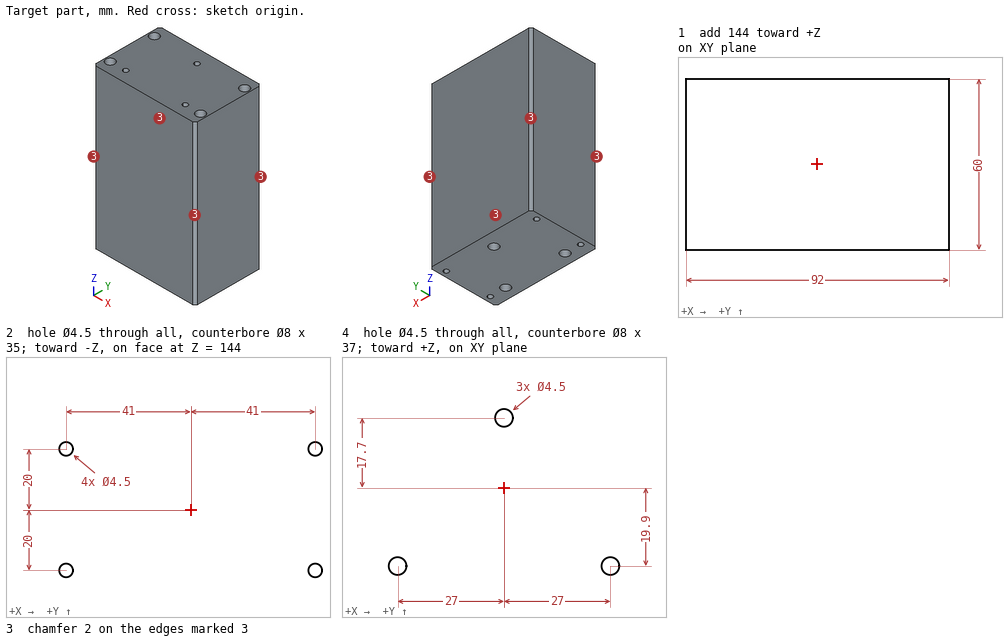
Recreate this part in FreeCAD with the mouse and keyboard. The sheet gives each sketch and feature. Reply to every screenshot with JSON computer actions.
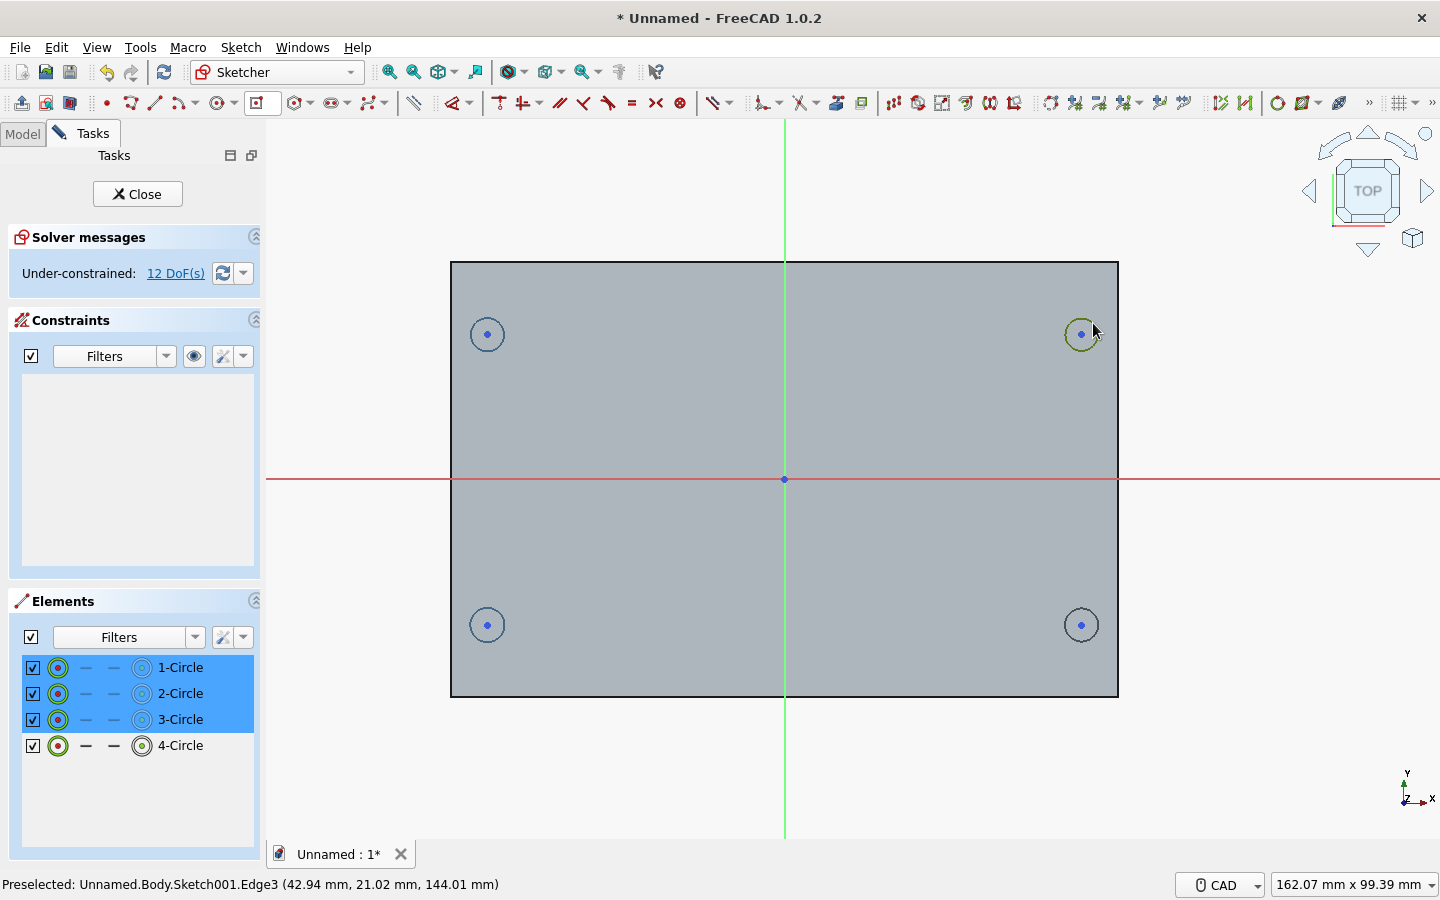
{"action": "left_click", "coordinate": [1093, 613]}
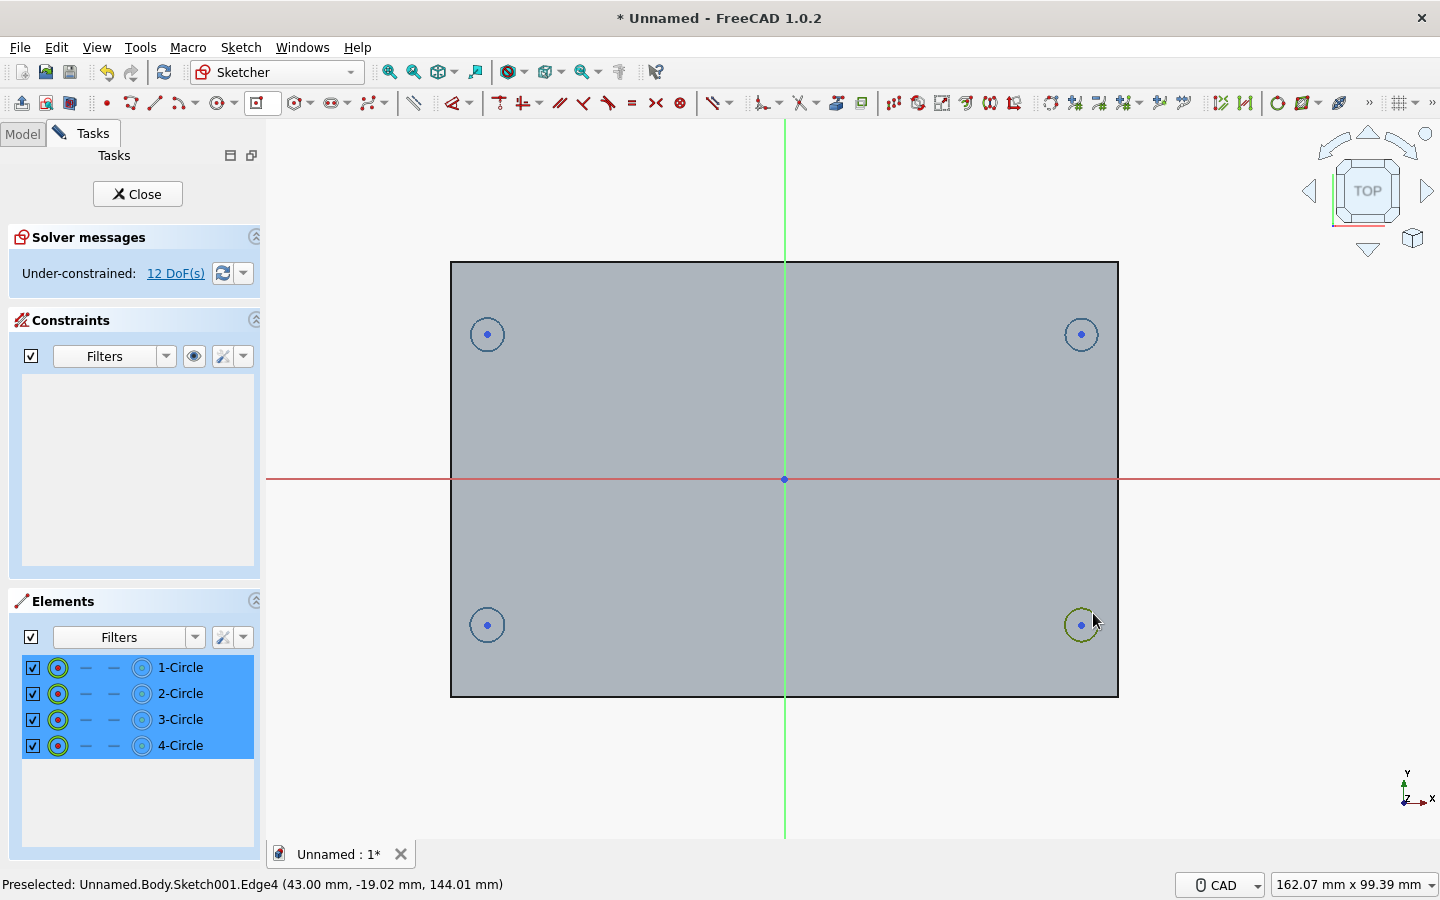
{"action": "left_click", "coordinate": [632, 104]}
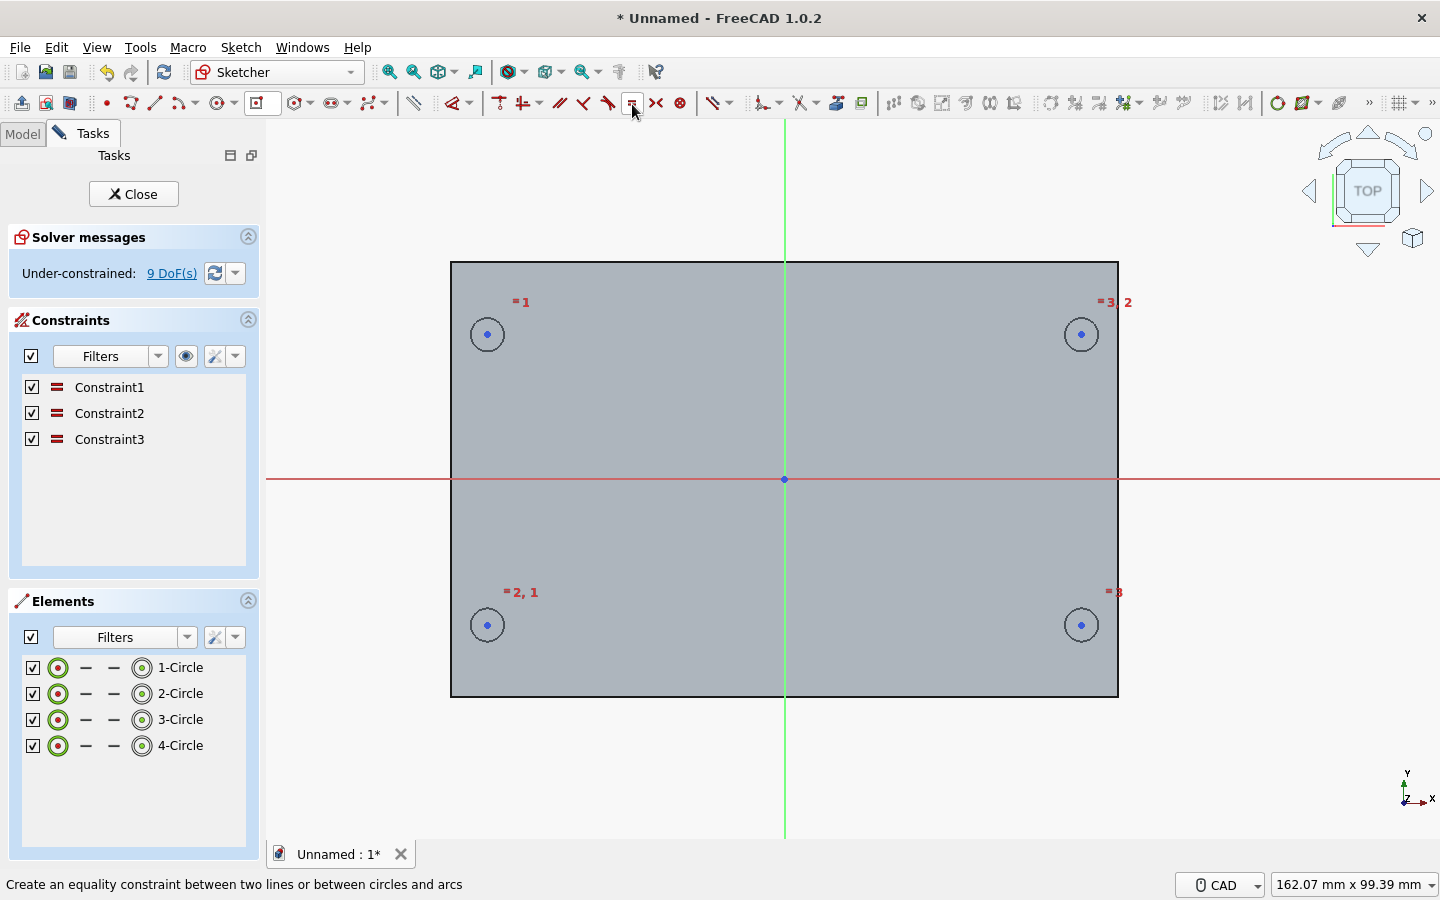
{"action": "left_click", "coordinate": [487, 335]}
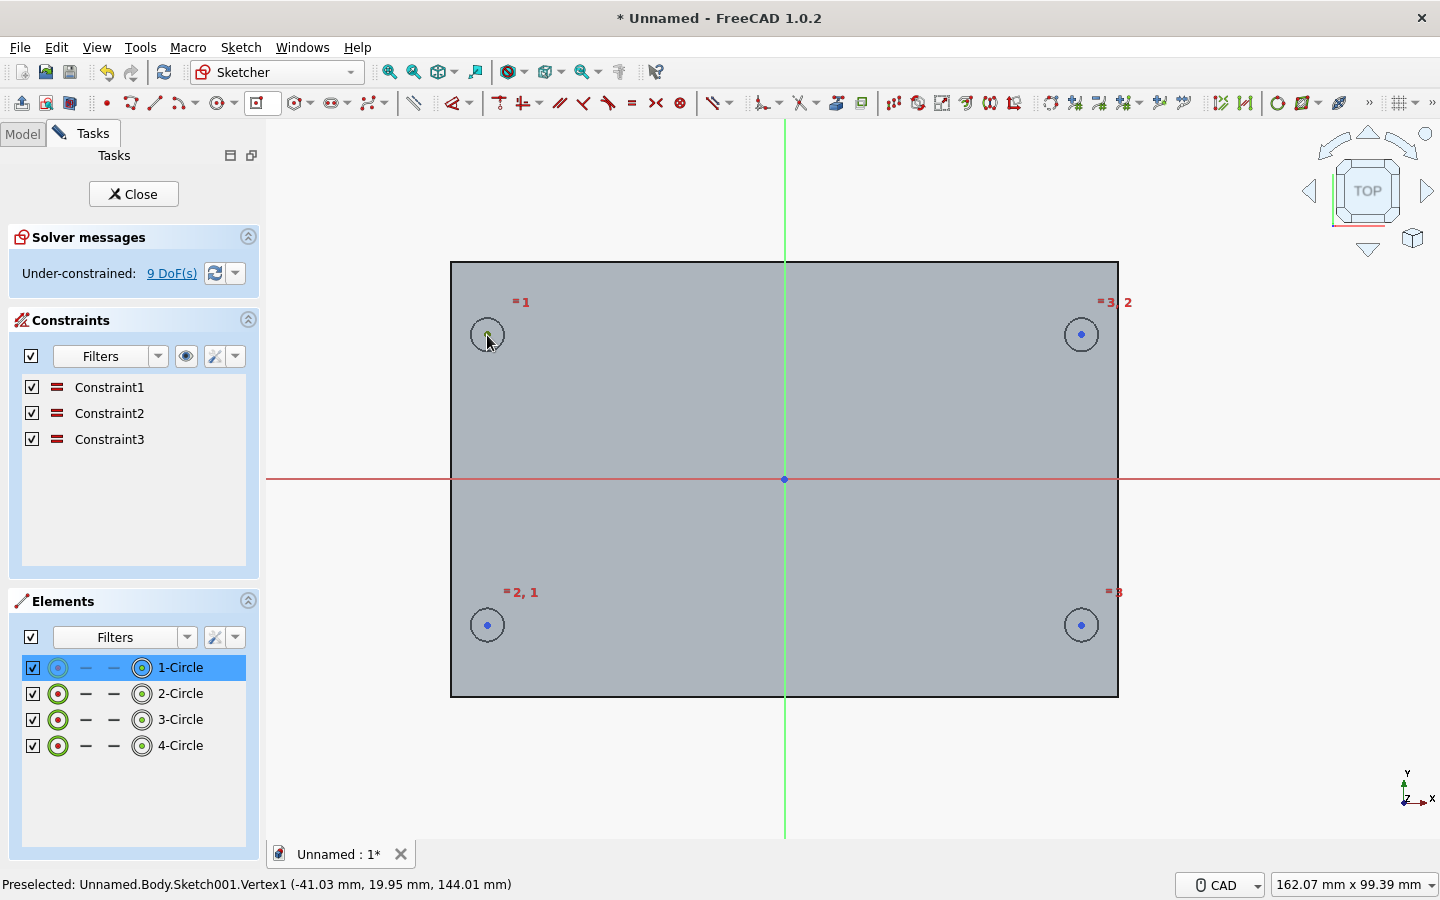
{"action": "left_click", "coordinate": [487, 625]}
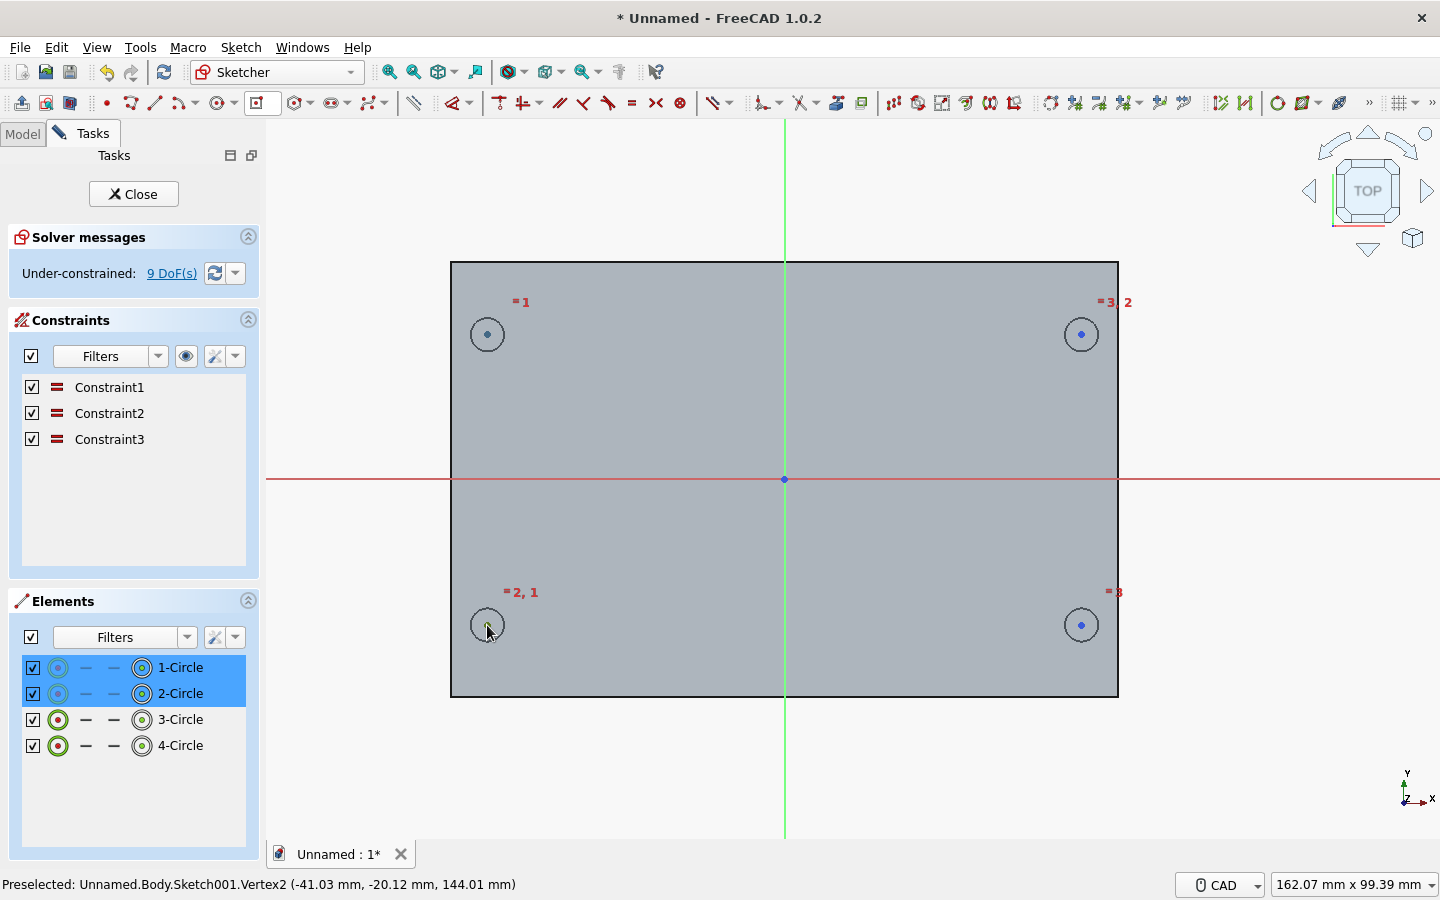
{"action": "left_click", "coordinate": [542, 104]}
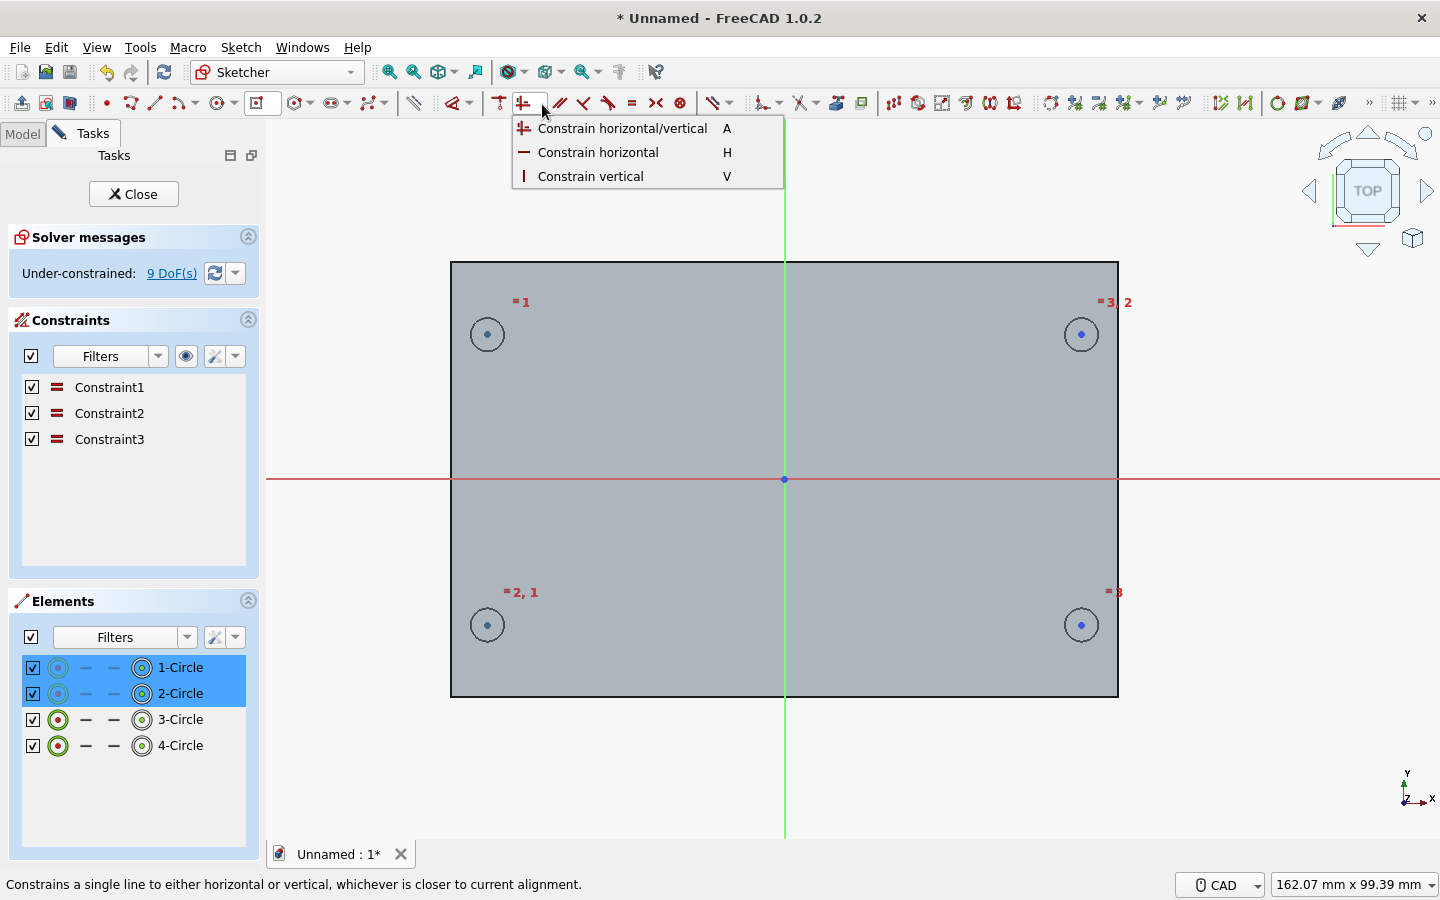
{"action": "left_click", "coordinate": [648, 176]}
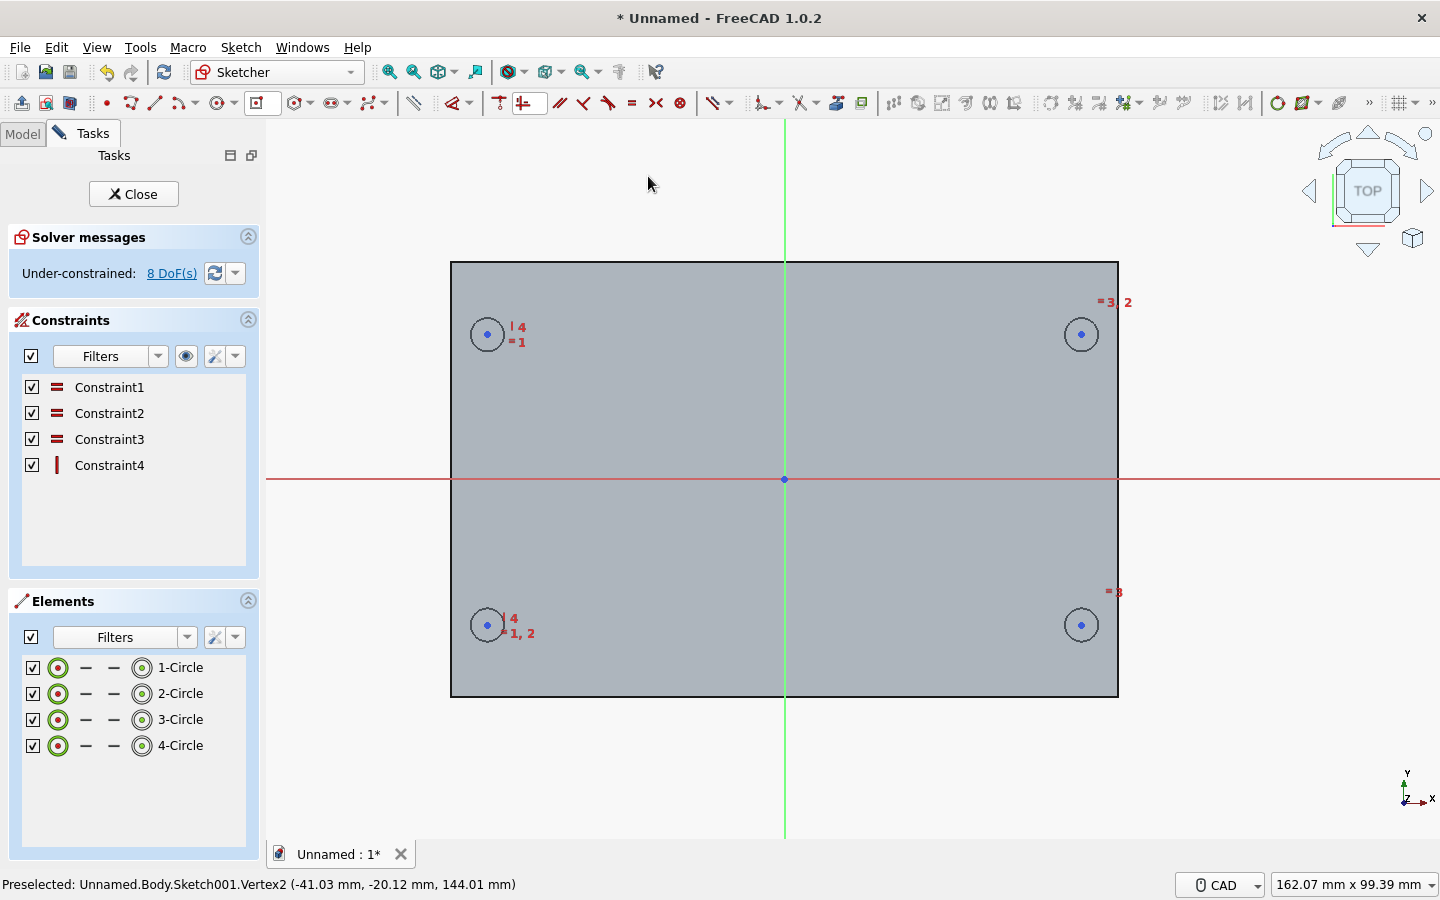
{"action": "left_click", "coordinate": [487, 335]}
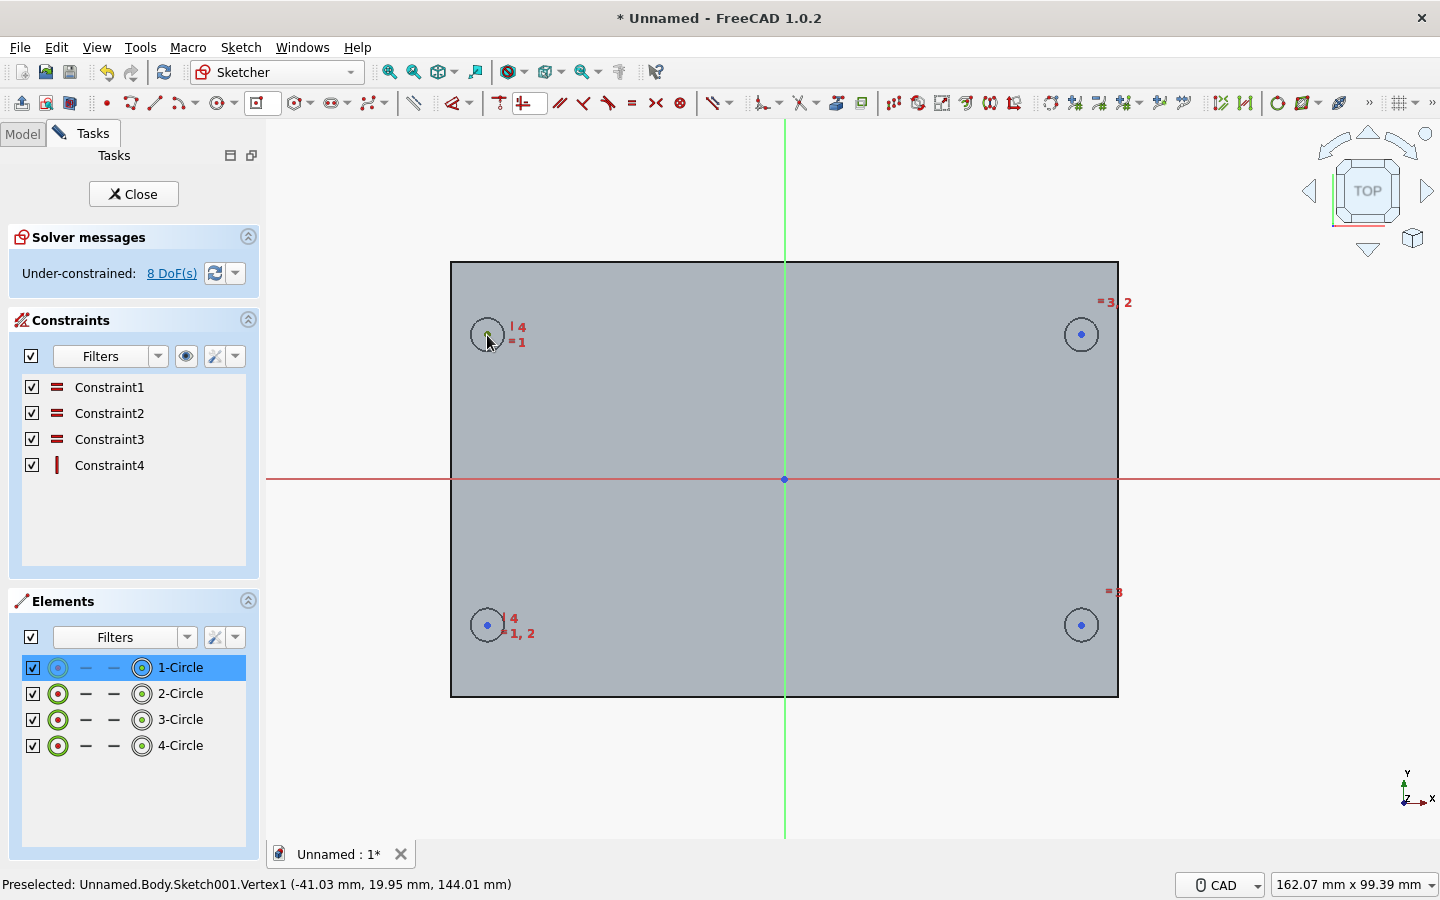
{"action": "left_click", "coordinate": [1082, 335]}